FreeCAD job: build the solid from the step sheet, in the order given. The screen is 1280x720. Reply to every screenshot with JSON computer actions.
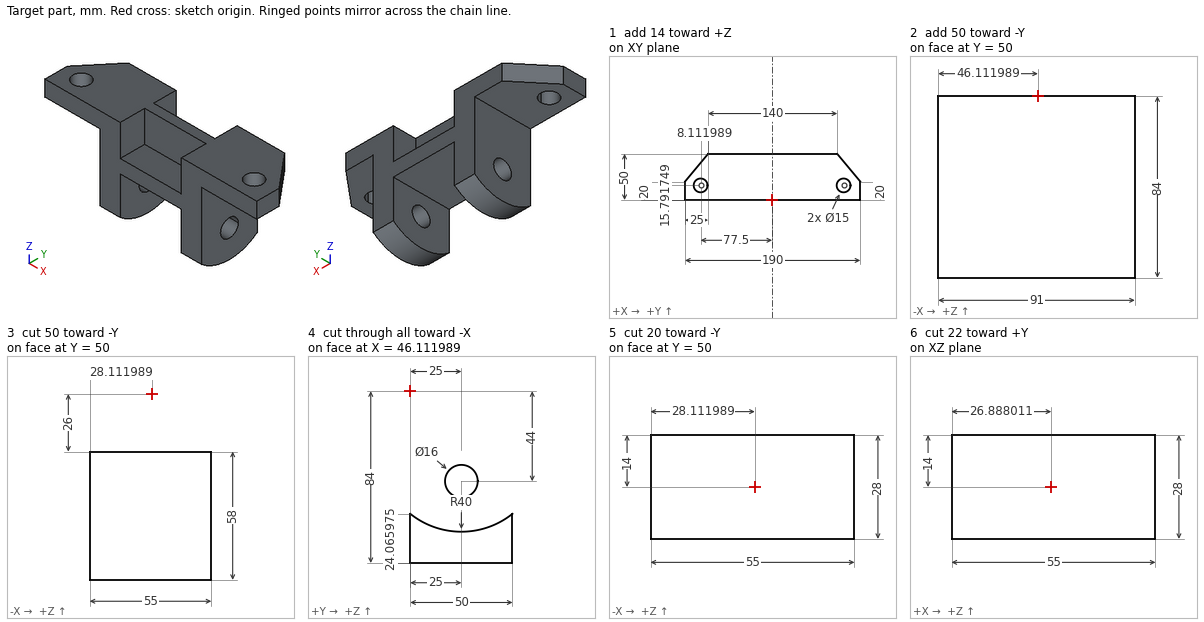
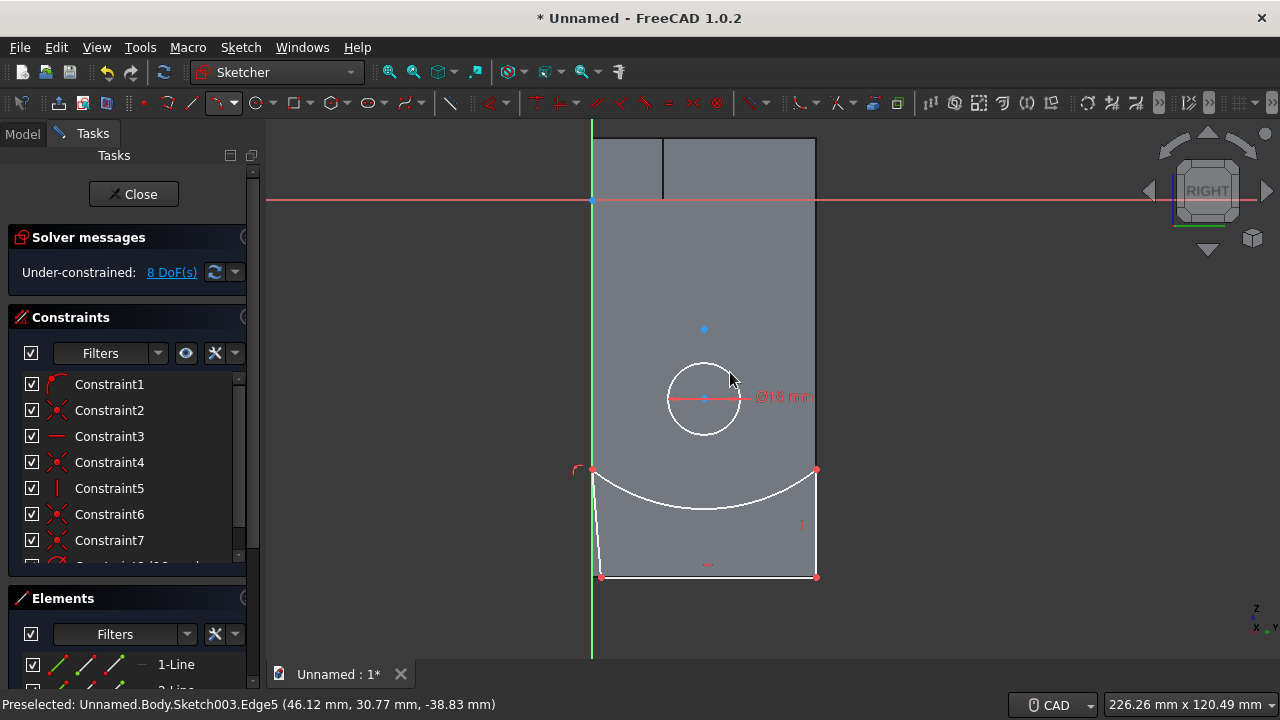
{"action": "left_click", "coordinate": [595, 502]}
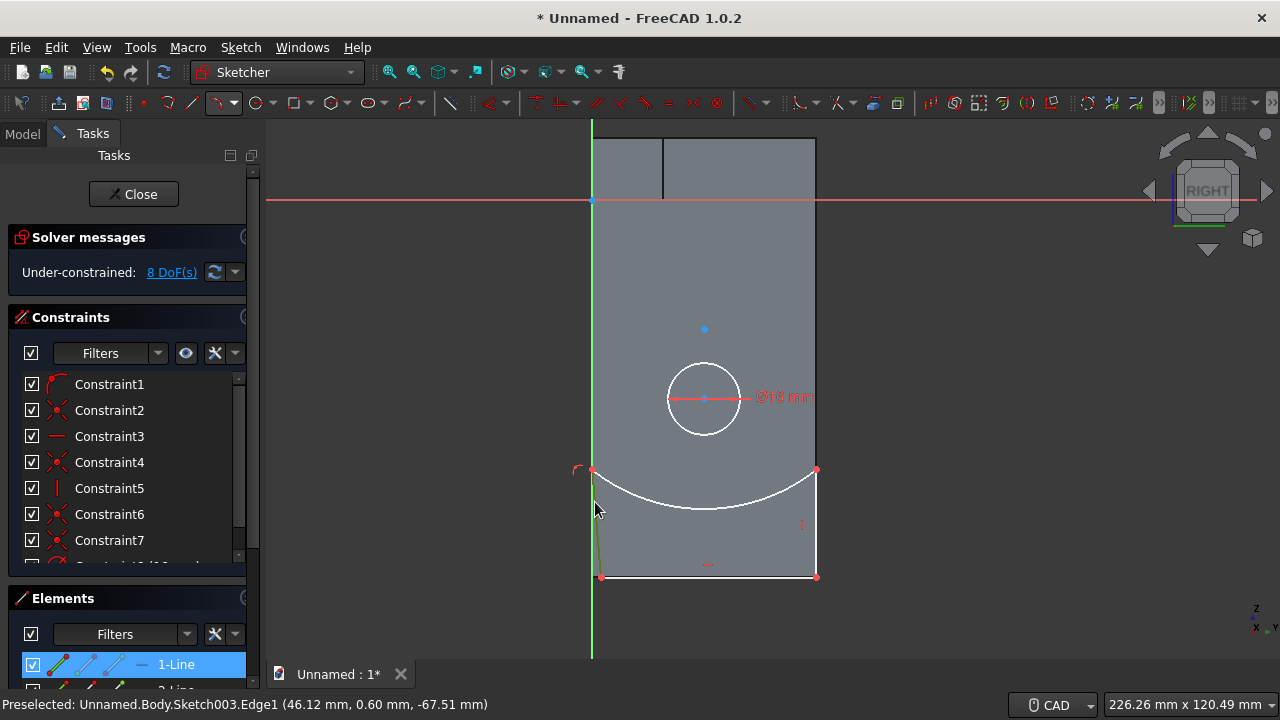
{"action": "key", "text": "v"}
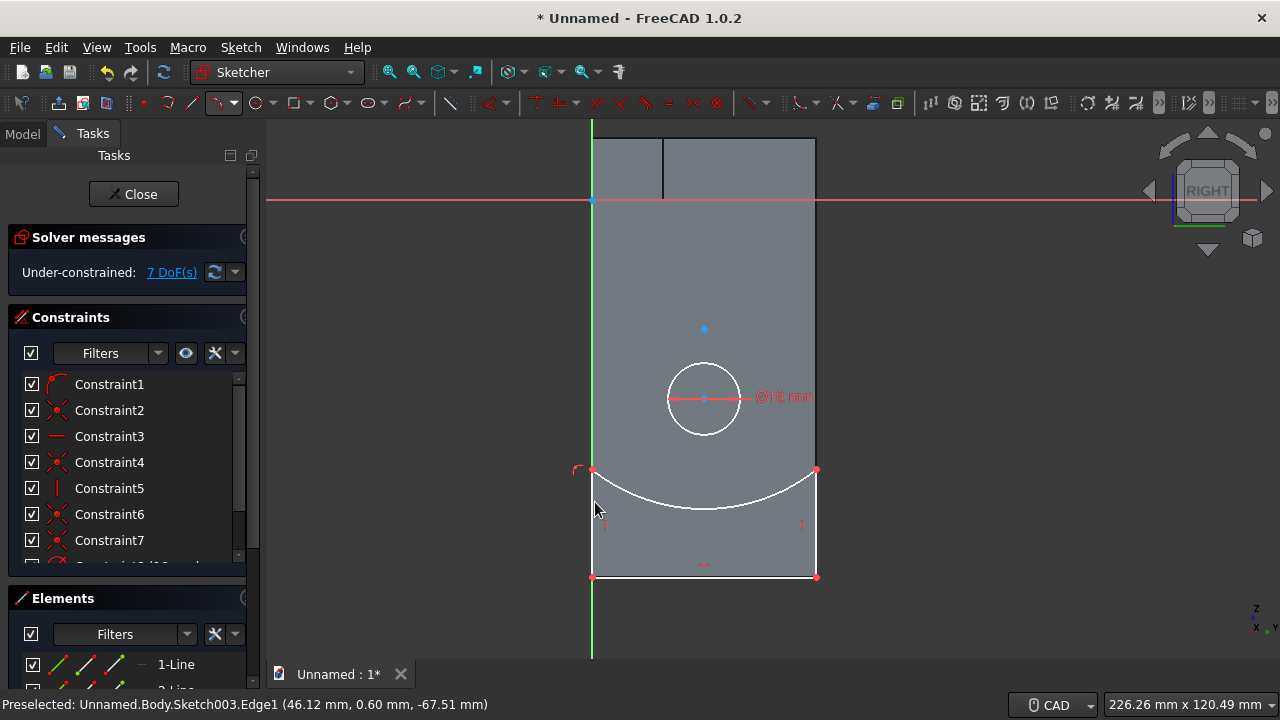
{"action": "left_click", "coordinate": [490, 104]}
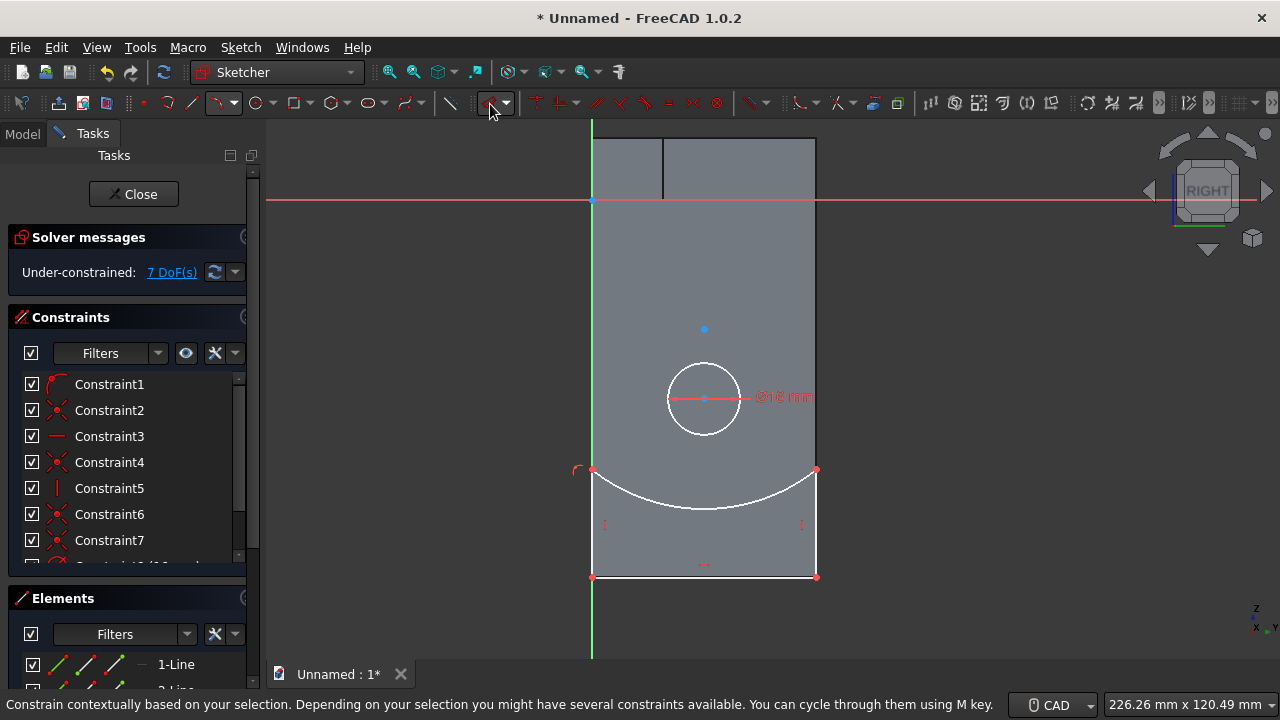
{"action": "left_click", "coordinate": [656, 503]}
{"action": "left_click", "coordinate": [647, 534]}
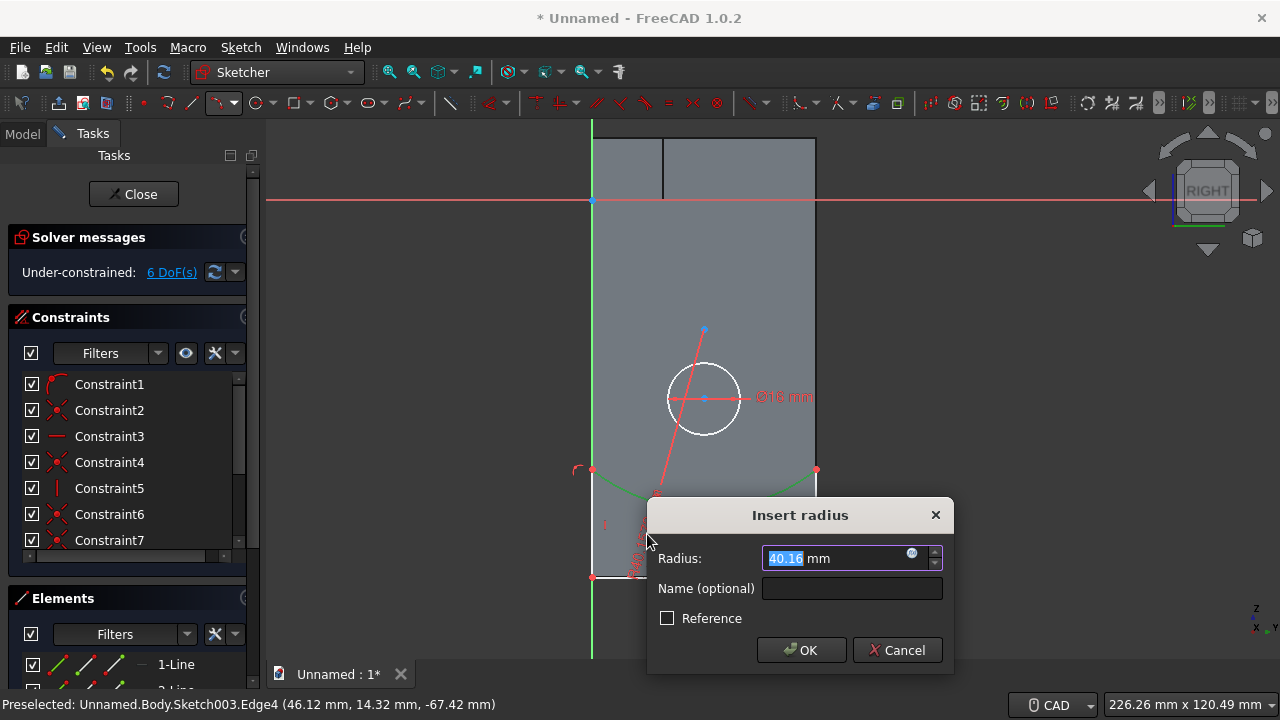
{"action": "type", "text": "40"}
{"action": "key", "text": "Return"}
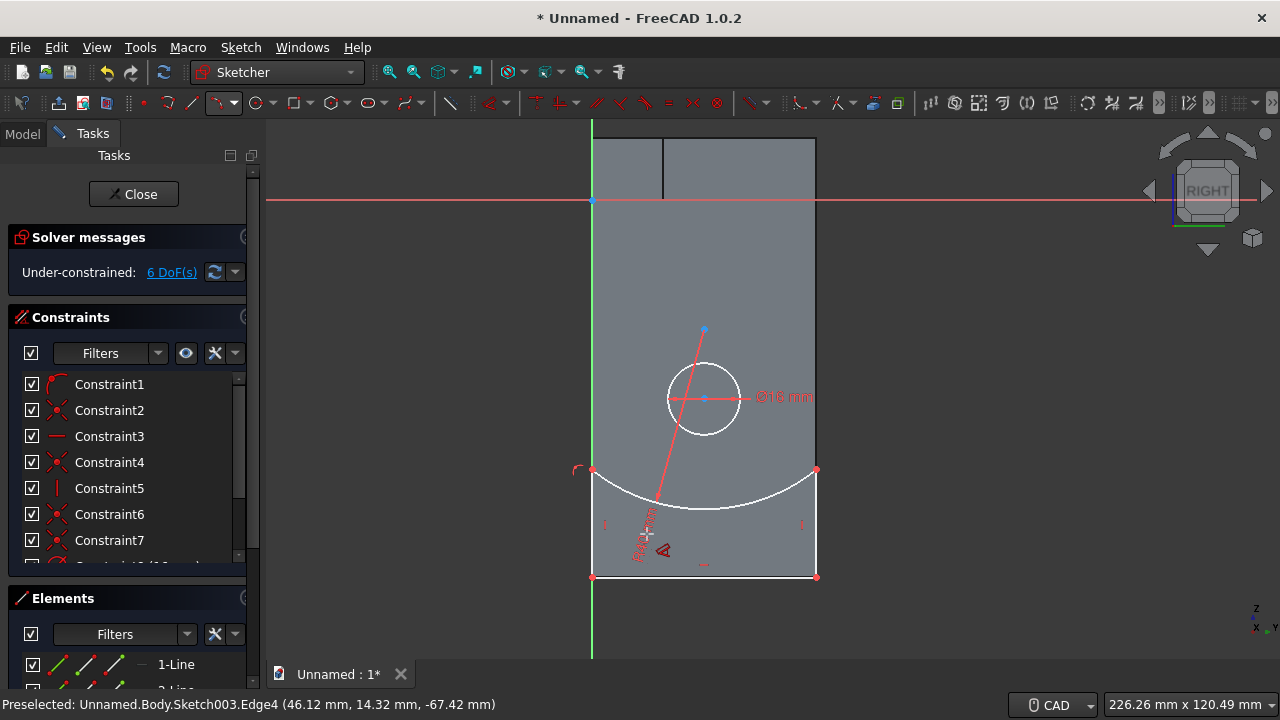
{"action": "left_click", "coordinate": [659, 578]}
{"action": "left_click", "coordinate": [704, 612]}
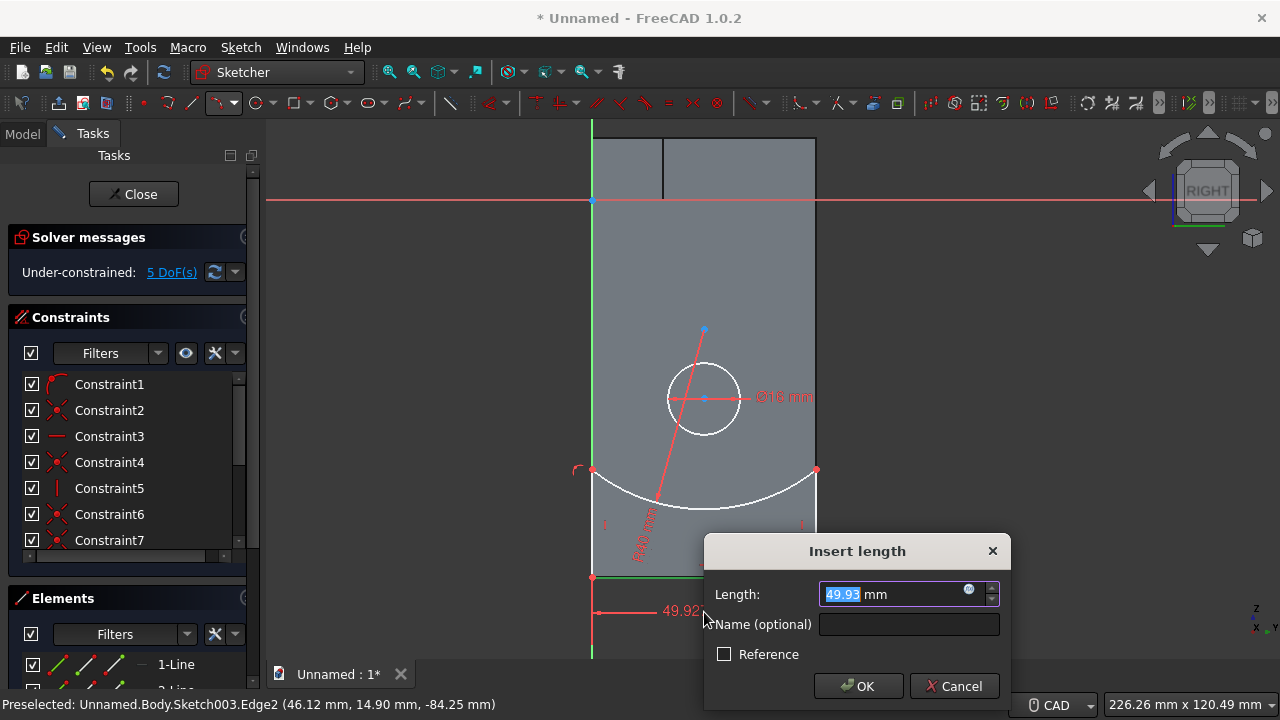
{"action": "type", "text": "50"}
{"action": "key", "text": "Return"}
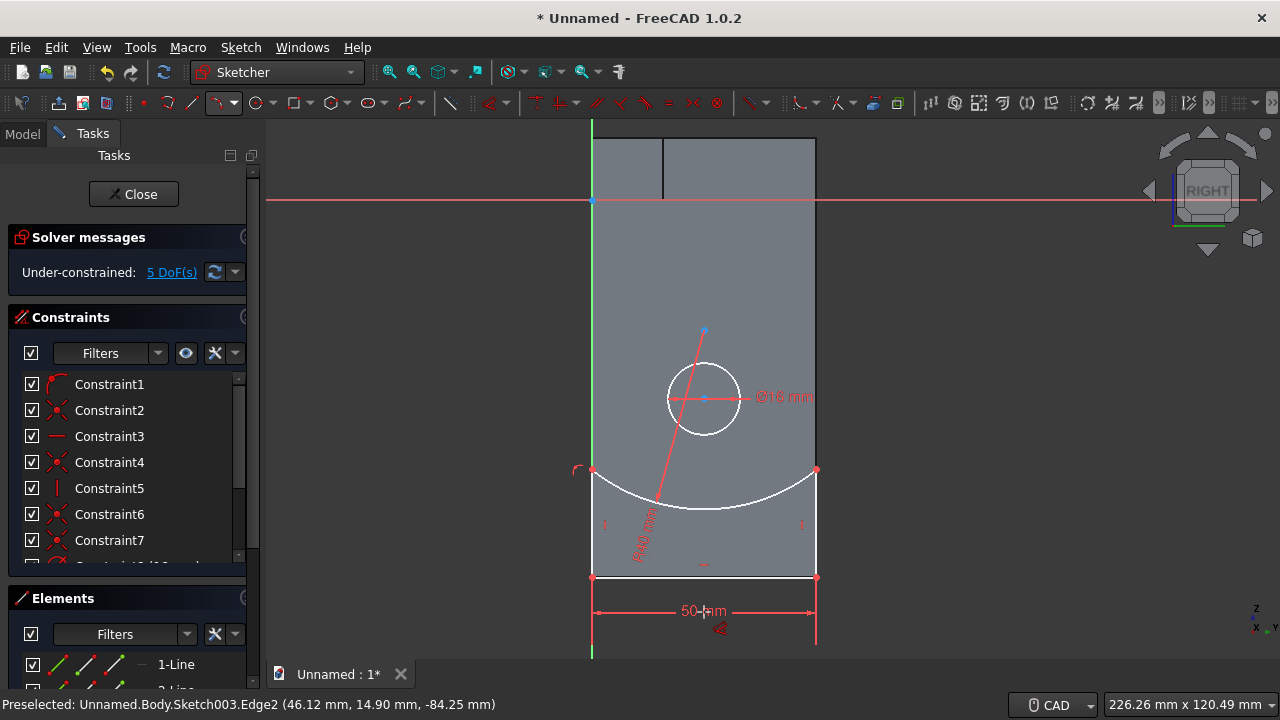
{"action": "left_click", "coordinate": [704, 399]}
{"action": "left_click", "coordinate": [648, 166]}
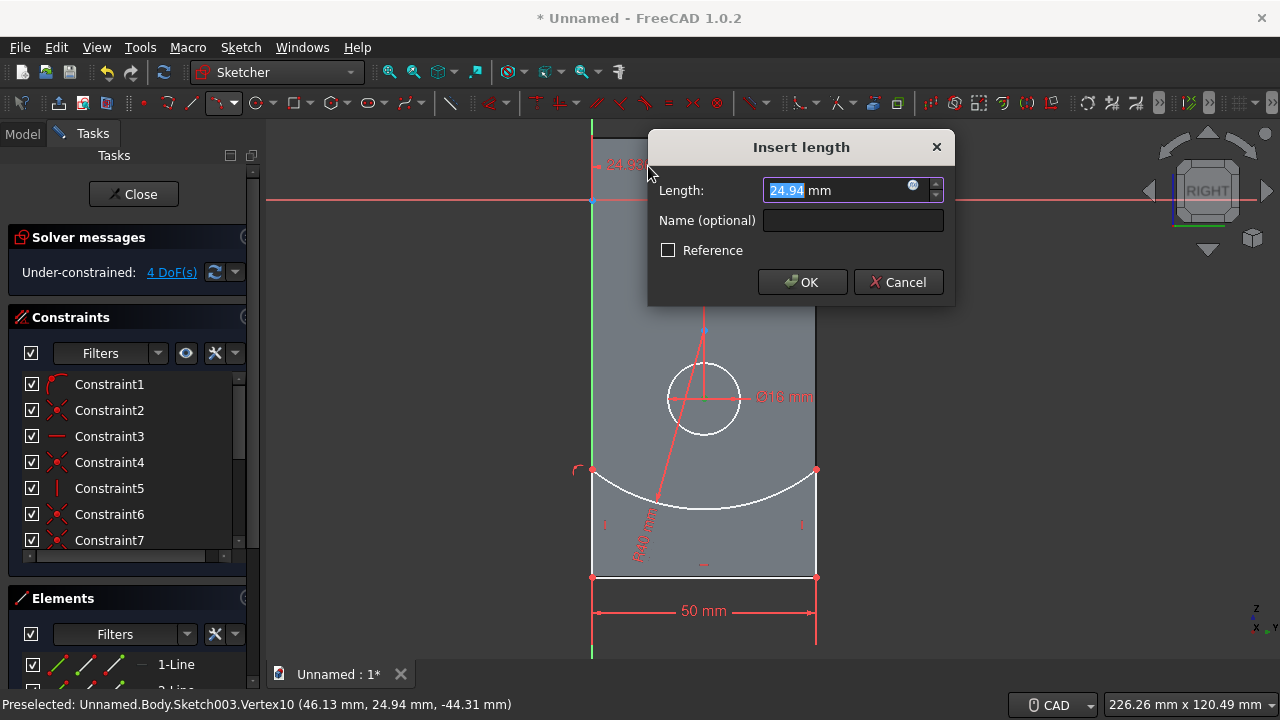
{"action": "type", "text": "25"}
{"action": "key", "text": "Return"}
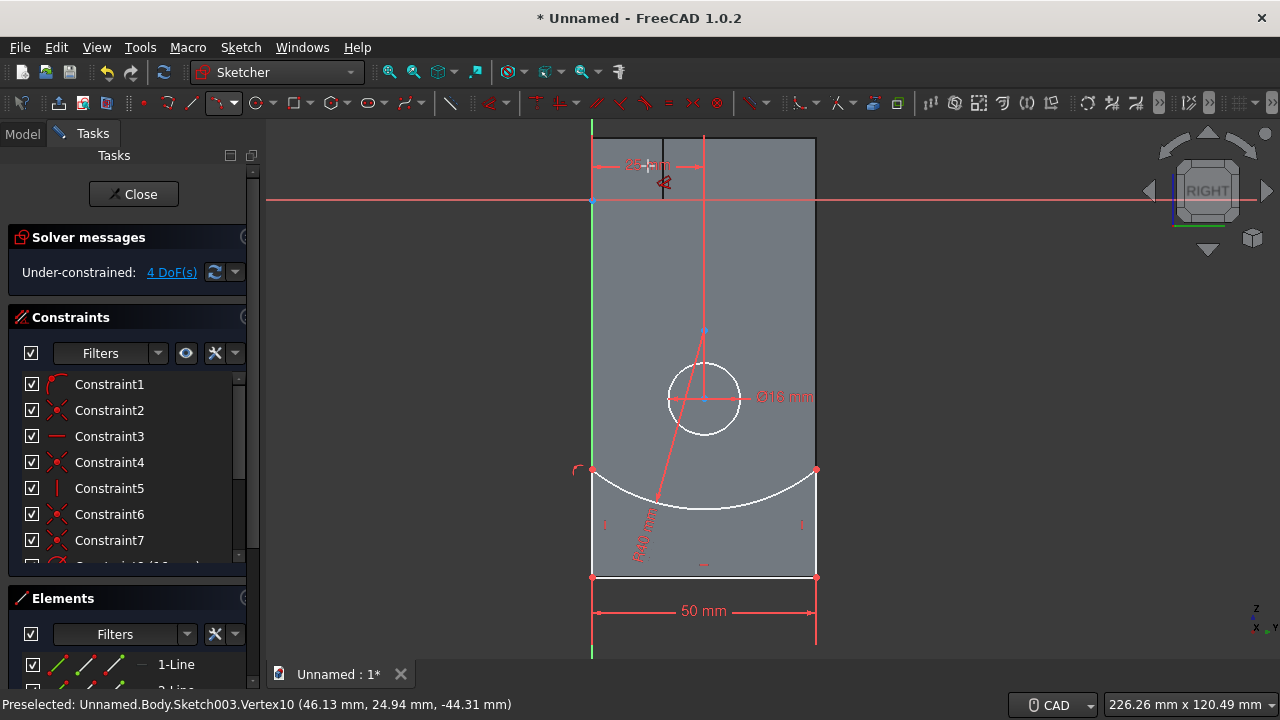
{"action": "left_click", "coordinate": [704, 399]}
{"action": "left_click", "coordinate": [558, 300]}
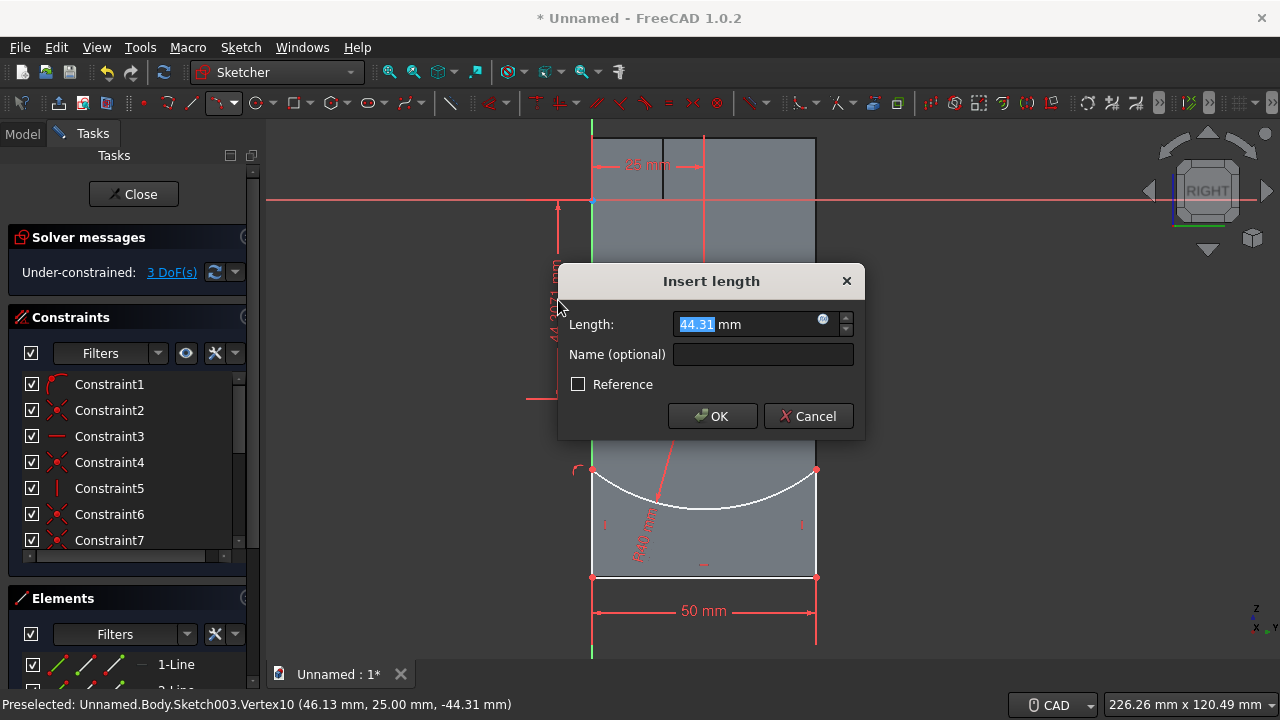
{"action": "type", "text": "44"}
{"action": "key", "text": "Return"}